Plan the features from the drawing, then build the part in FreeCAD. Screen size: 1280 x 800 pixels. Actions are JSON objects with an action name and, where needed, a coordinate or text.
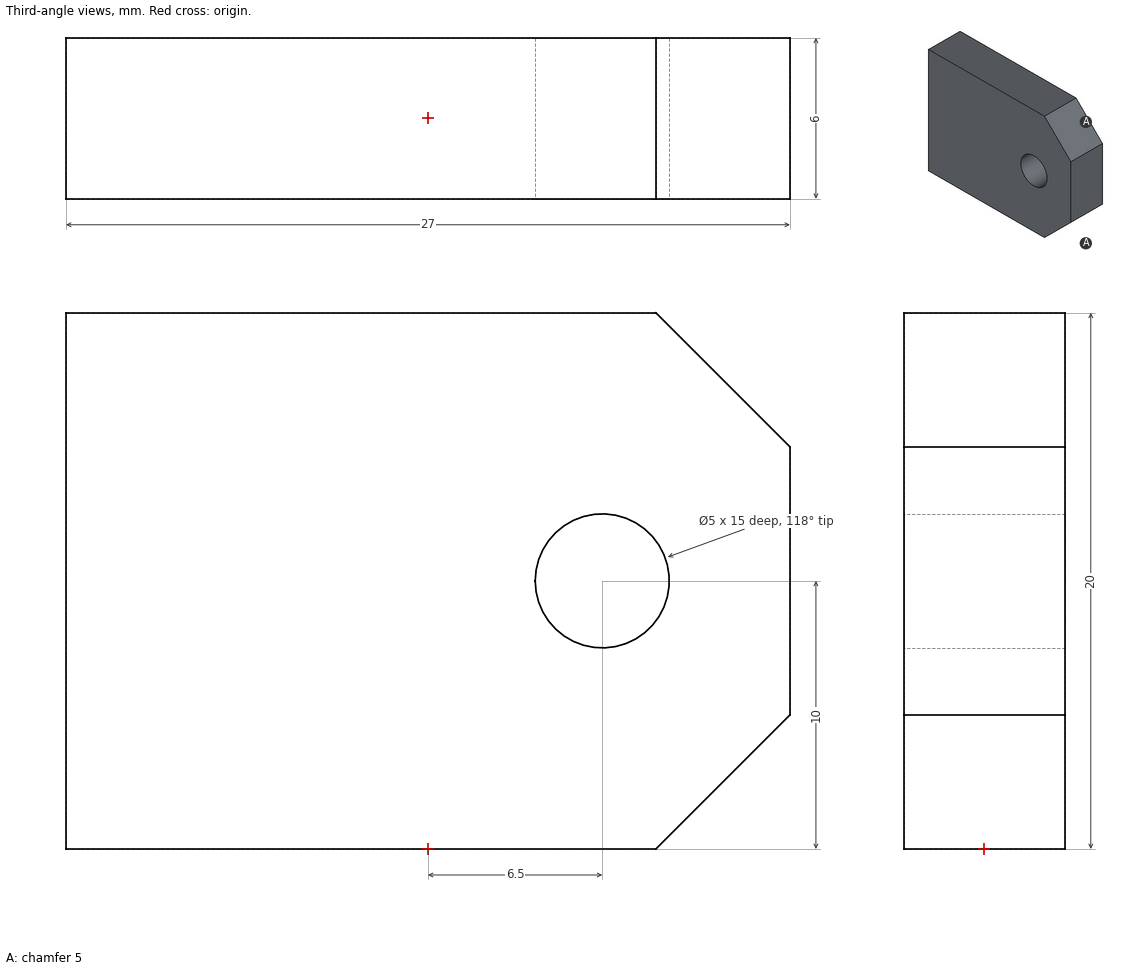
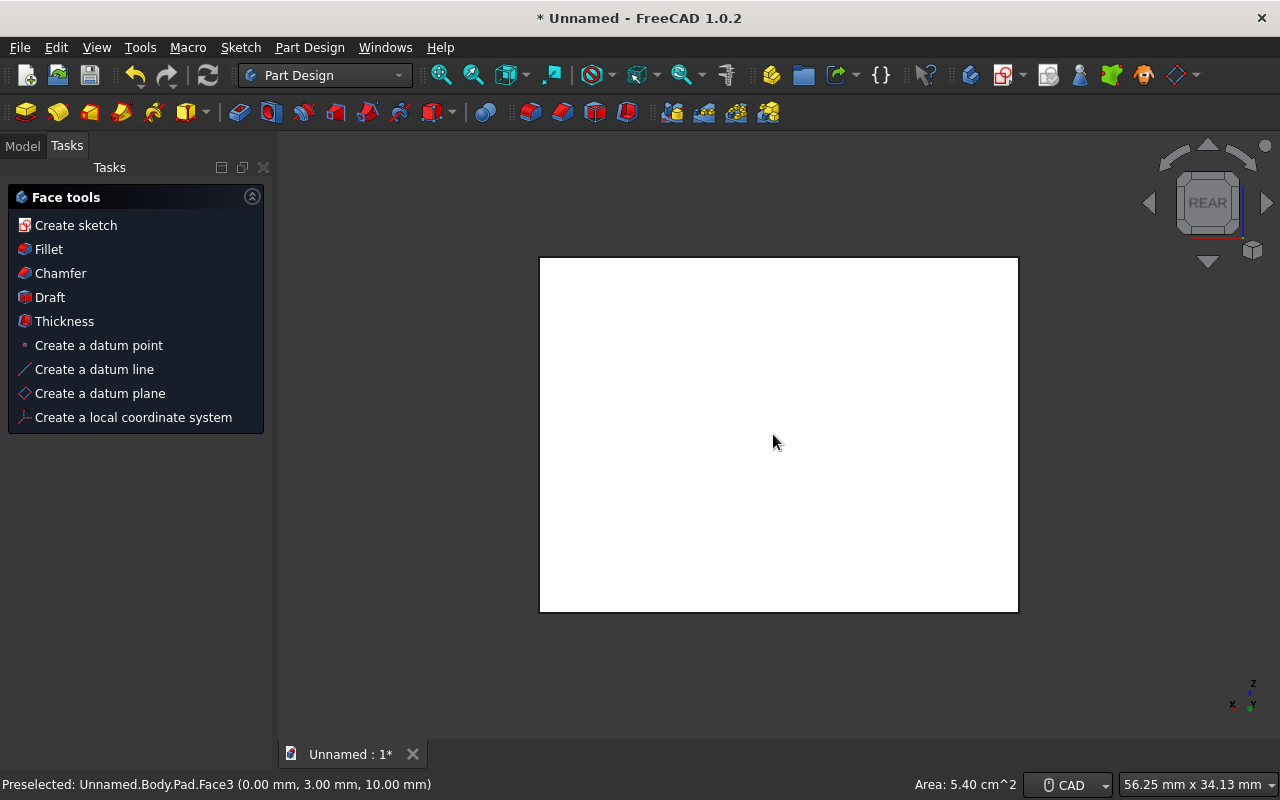
{"action": "left_click", "coordinate": [1004, 76]}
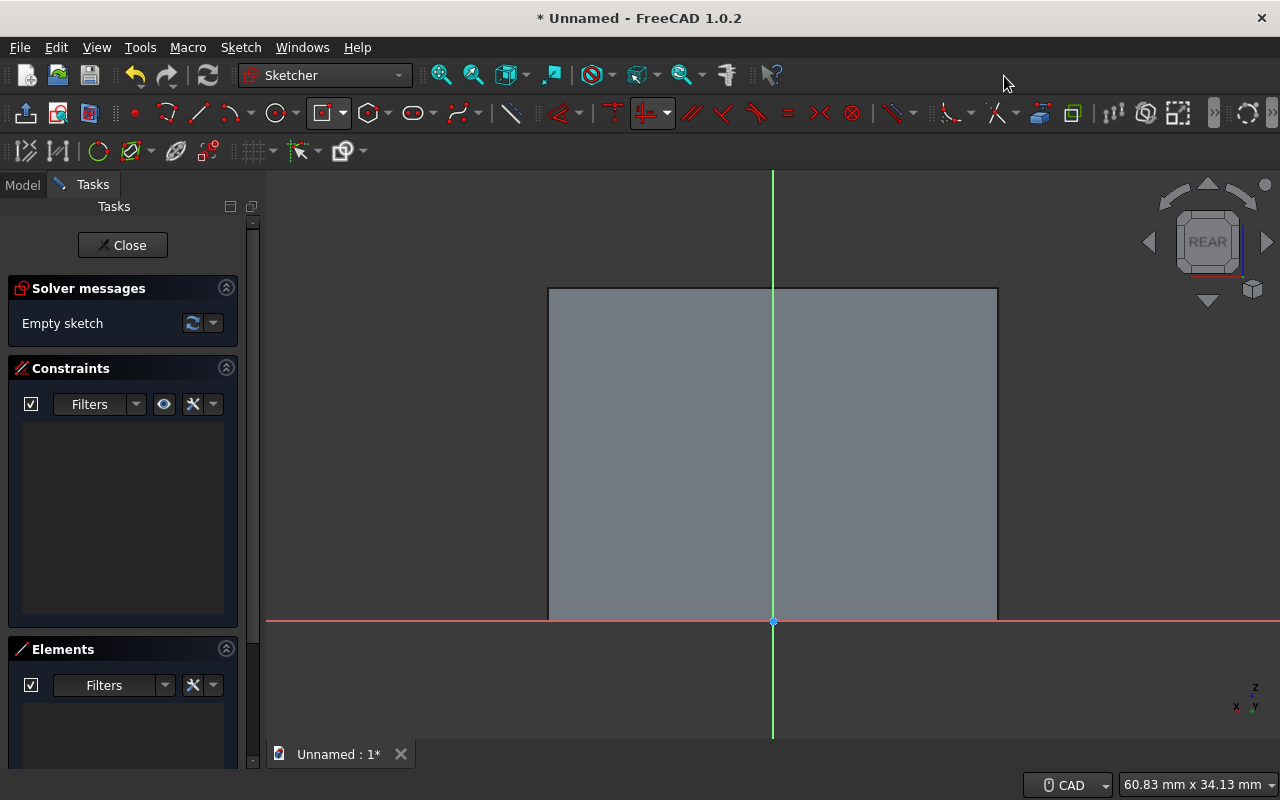
{"action": "scroll", "coordinate": [652, 454], "scroll_direction": "up", "scroll_amount": 7}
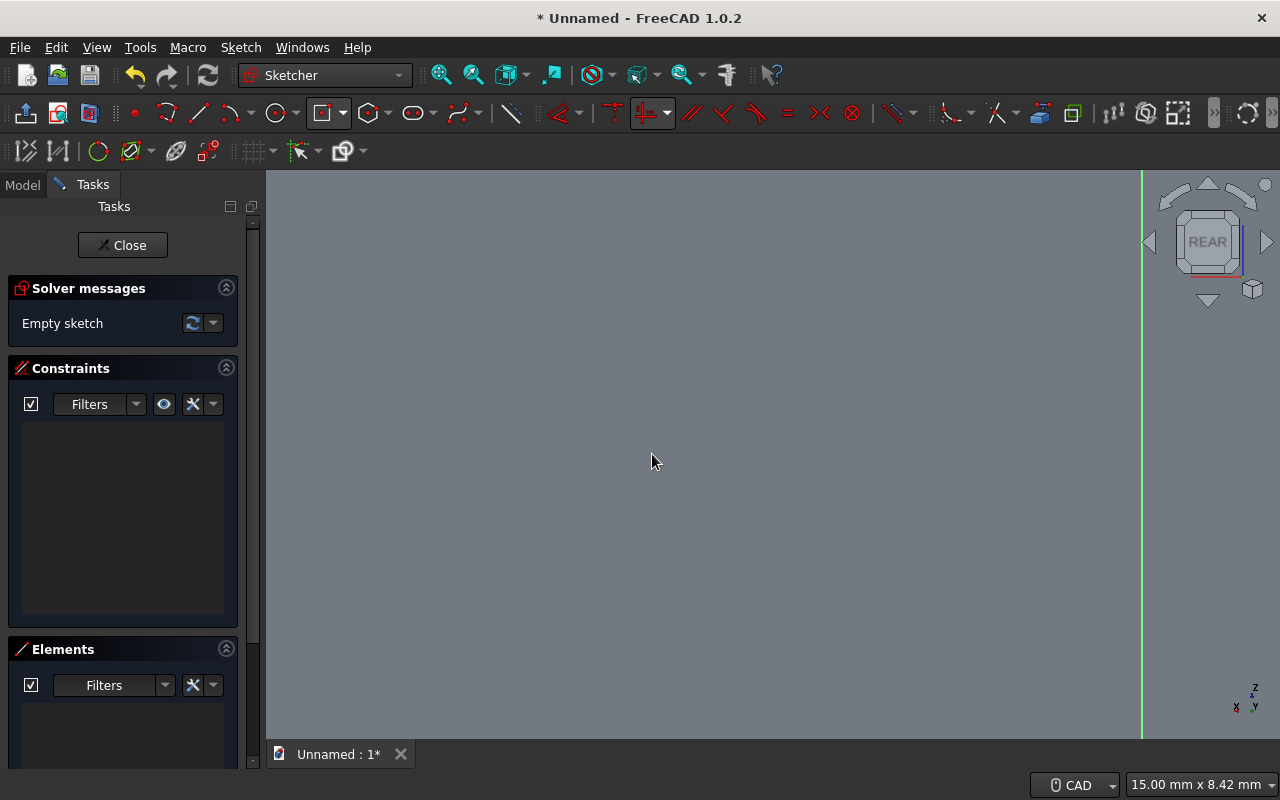
{"action": "left_click", "coordinate": [276, 114]}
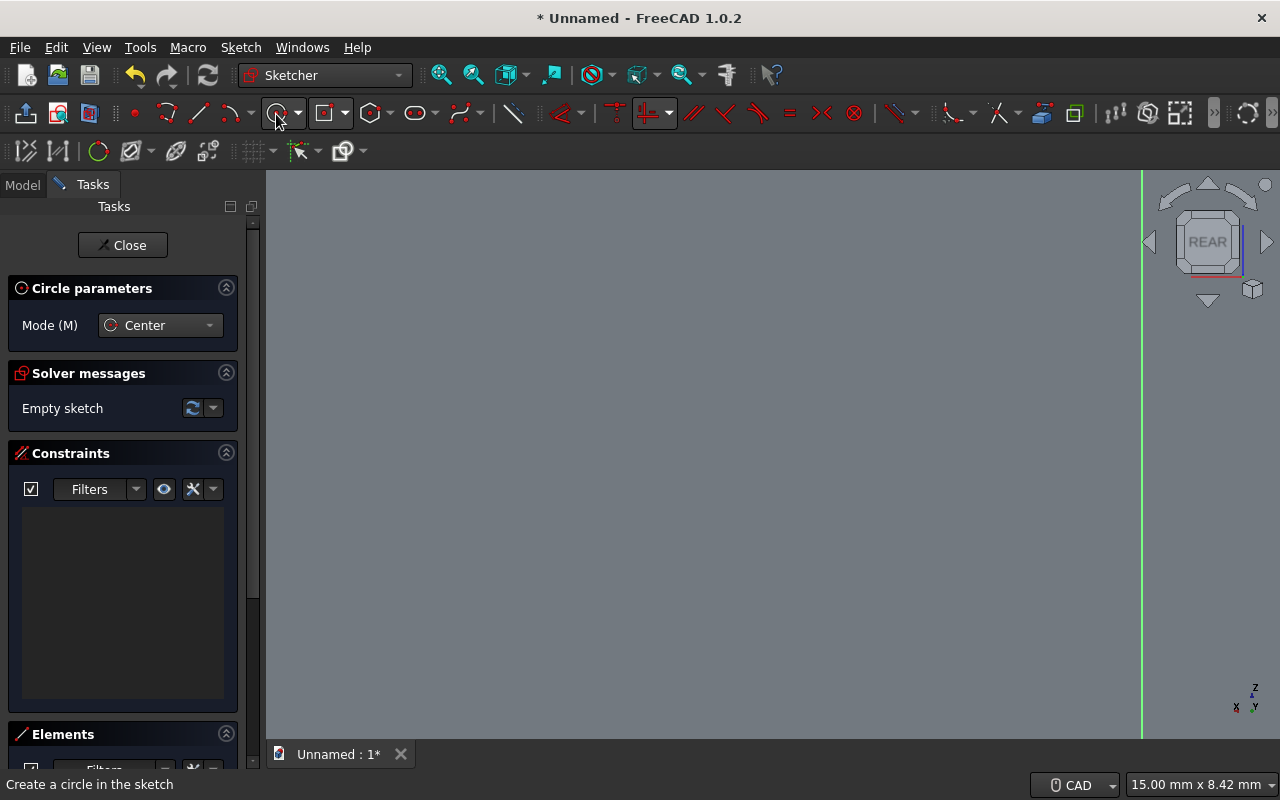
{"action": "left_click", "coordinate": [702, 454]}
{"action": "left_click", "coordinate": [822, 335]}
{"action": "key", "text": "Escape"}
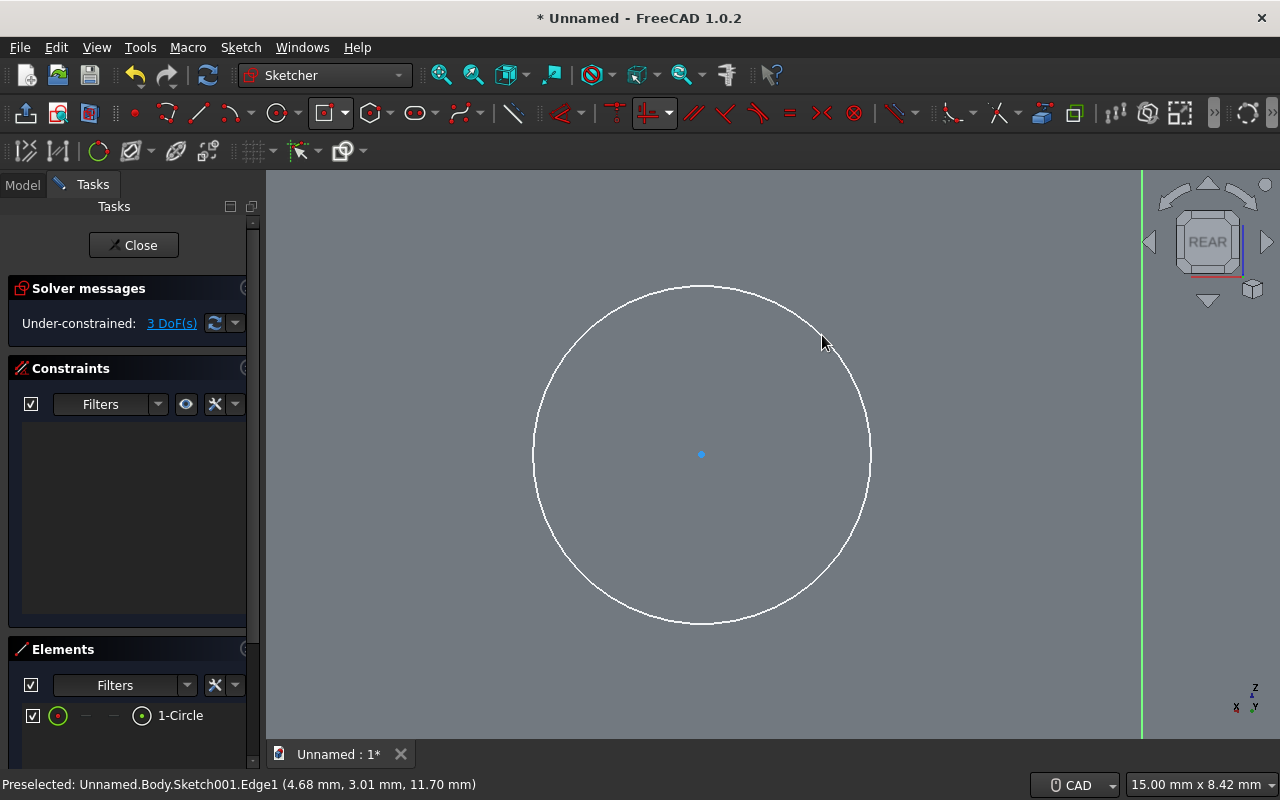
{"action": "left_click", "coordinate": [560, 114]}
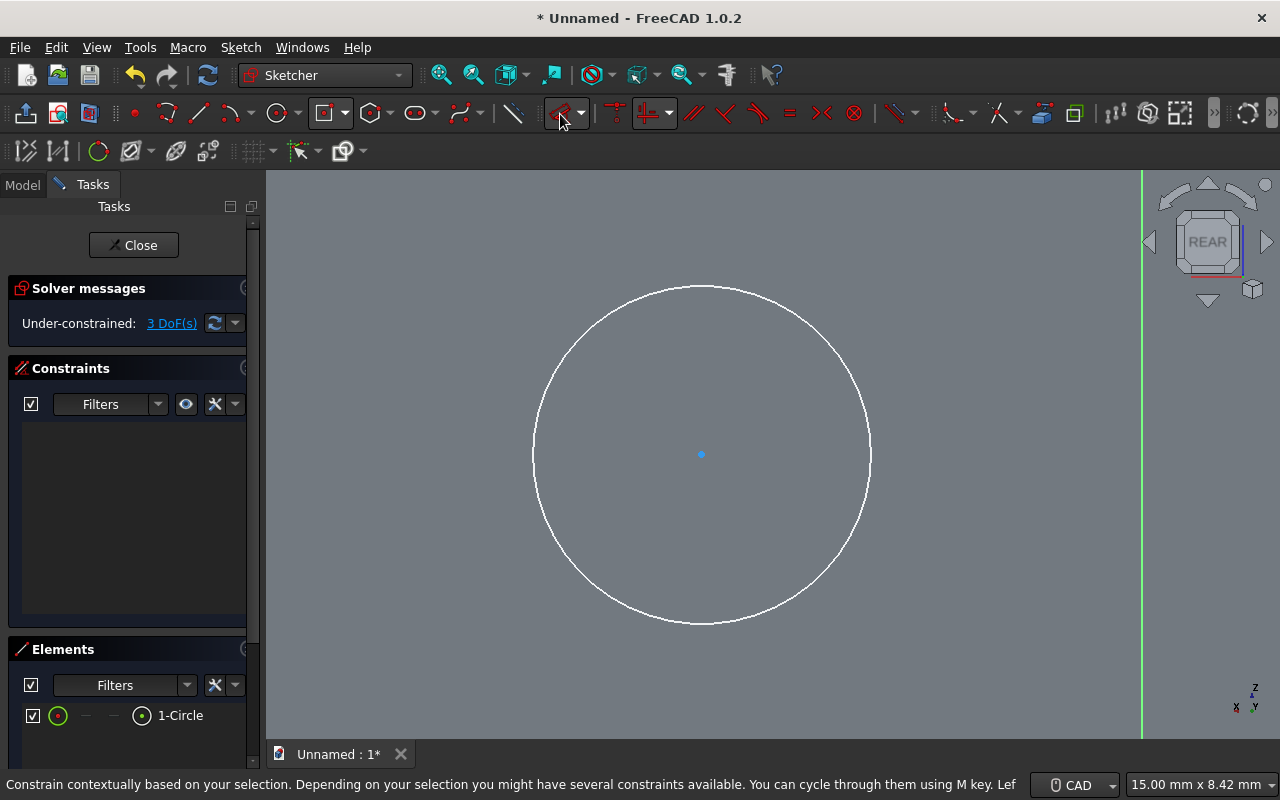
{"action": "left_click", "coordinate": [821, 335]}
{"action": "left_click", "coordinate": [844, 312]}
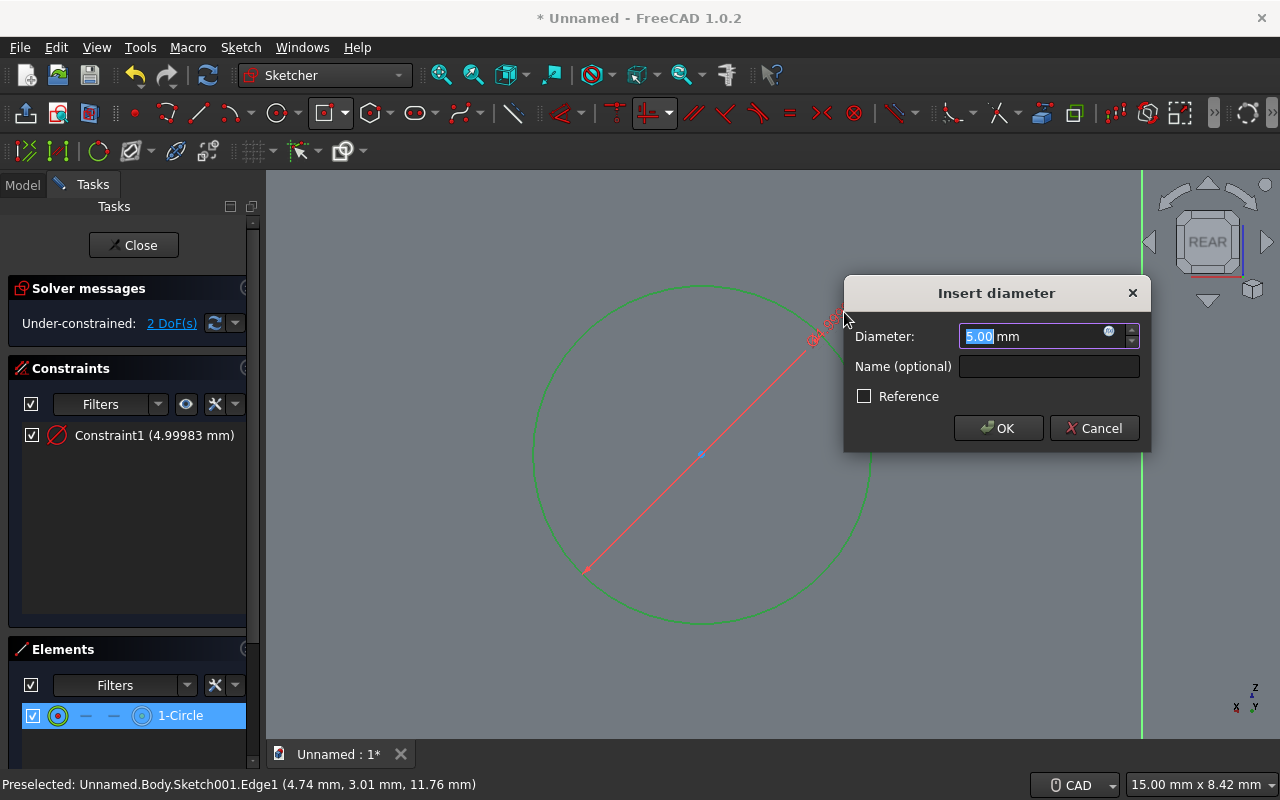
{"action": "type", "text": "5"}
{"action": "key", "text": "Return"}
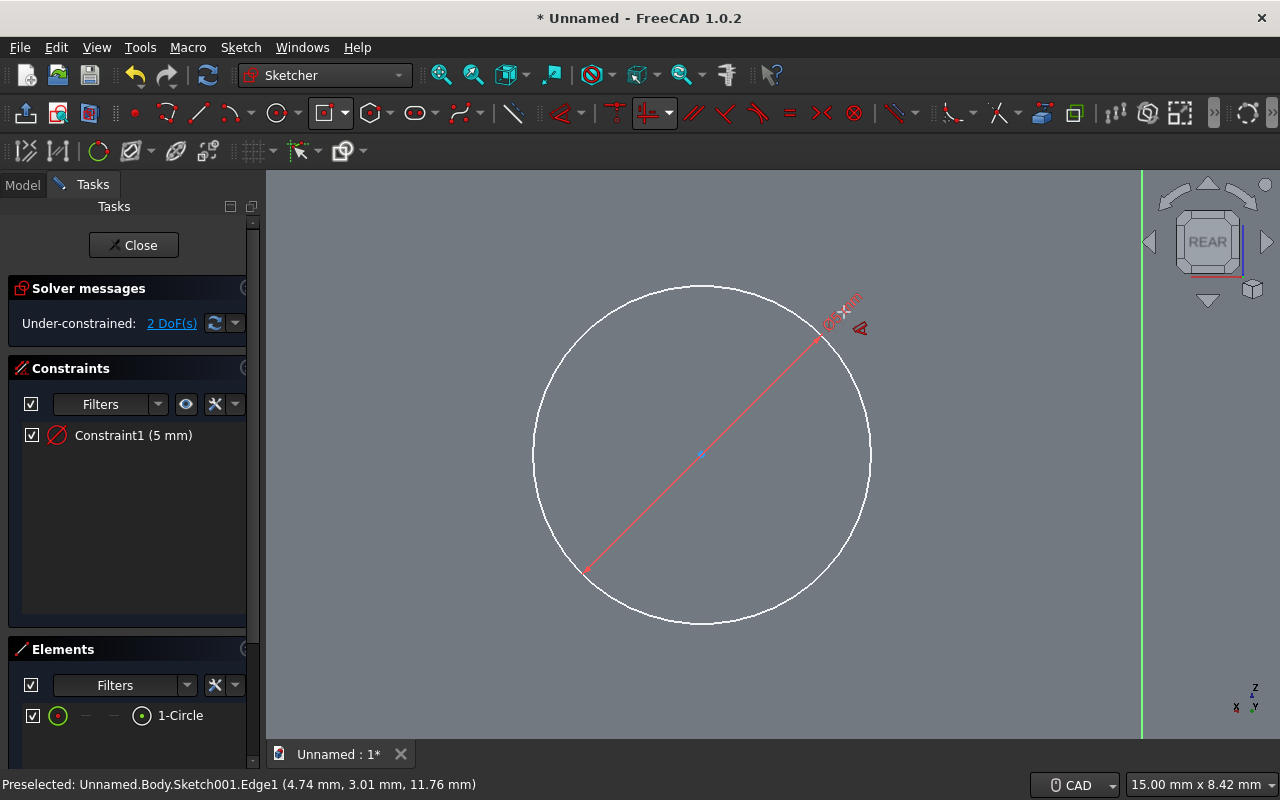
{"action": "left_click", "coordinate": [702, 455]}
{"action": "left_click", "coordinate": [668, 583]}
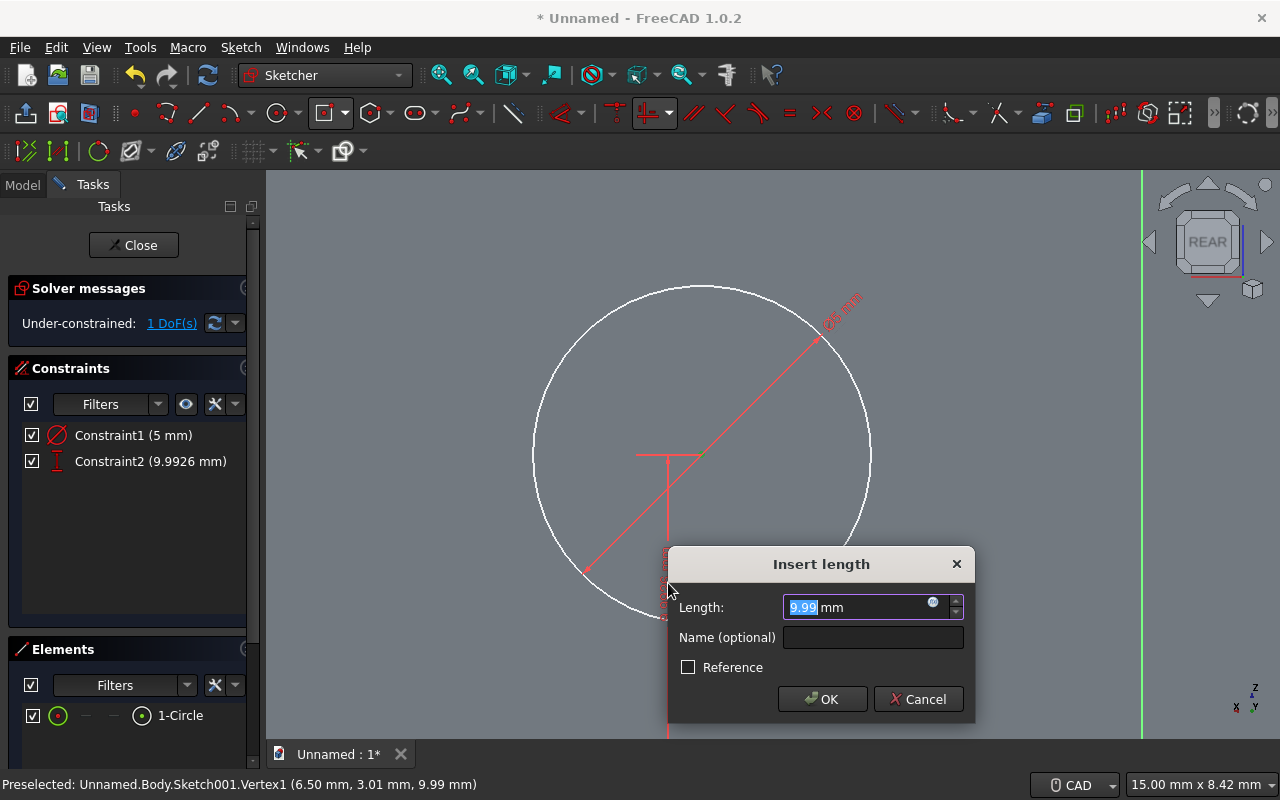
{"action": "type", "text": "10"}
{"action": "key", "text": "Return"}